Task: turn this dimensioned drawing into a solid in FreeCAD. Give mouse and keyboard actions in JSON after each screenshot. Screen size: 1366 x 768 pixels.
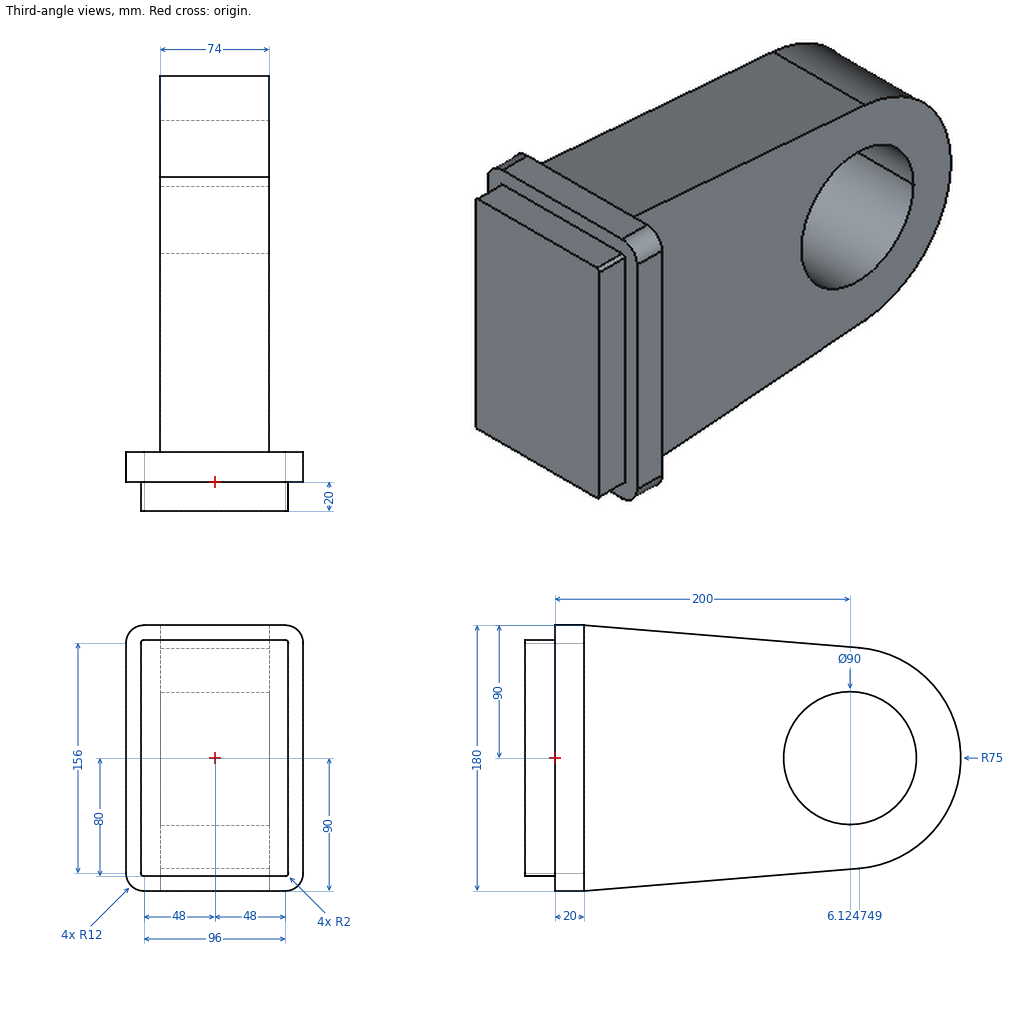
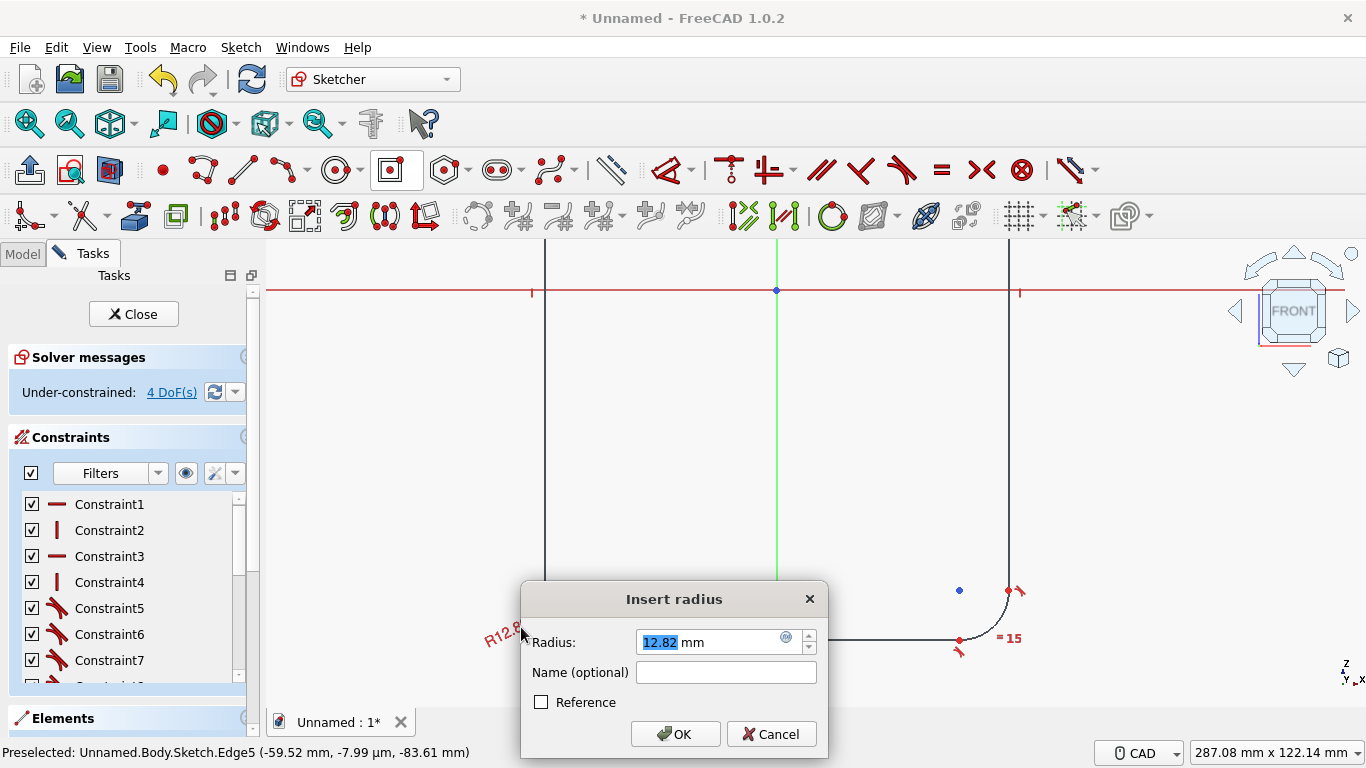
{"action": "type", "text": "12"}
{"action": "key", "text": "Return"}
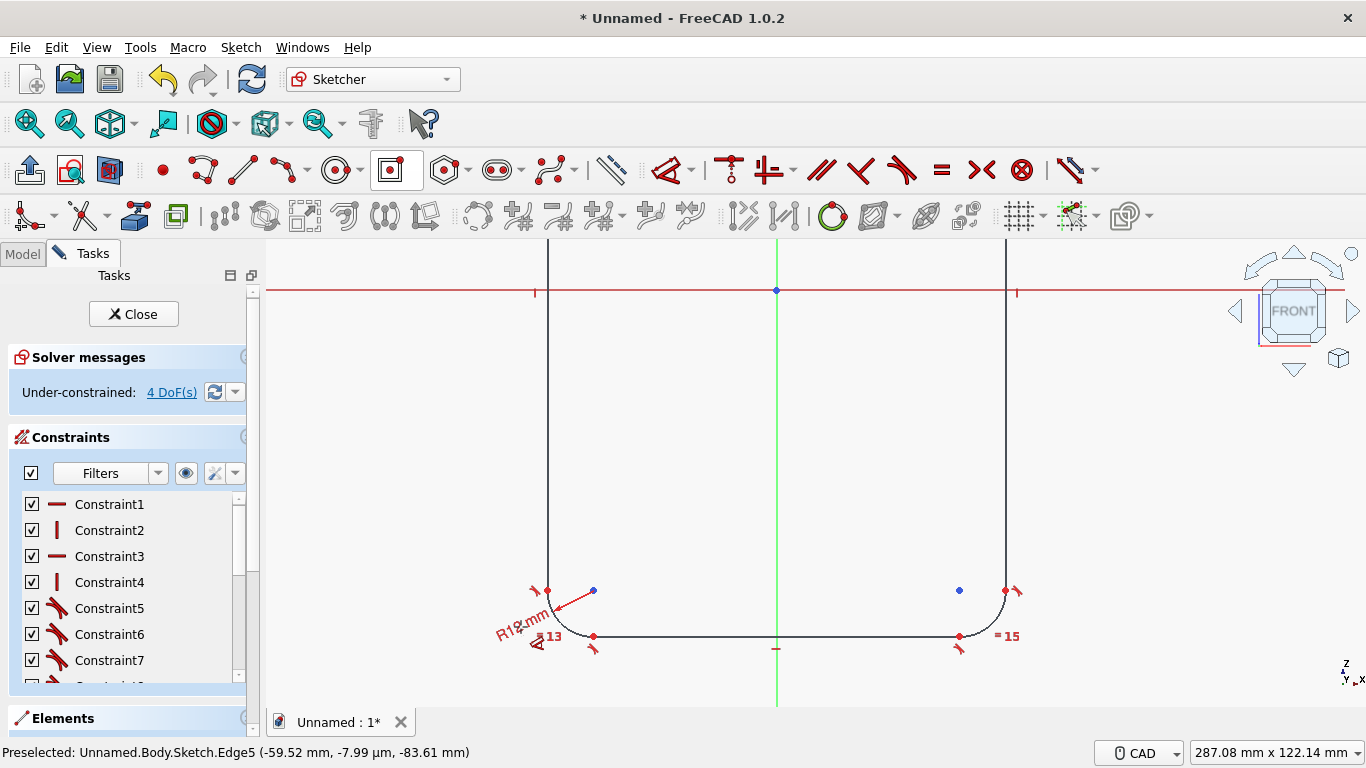
{"action": "left_click", "coordinate": [850, 637]}
{"action": "left_click", "coordinate": [692, 671]}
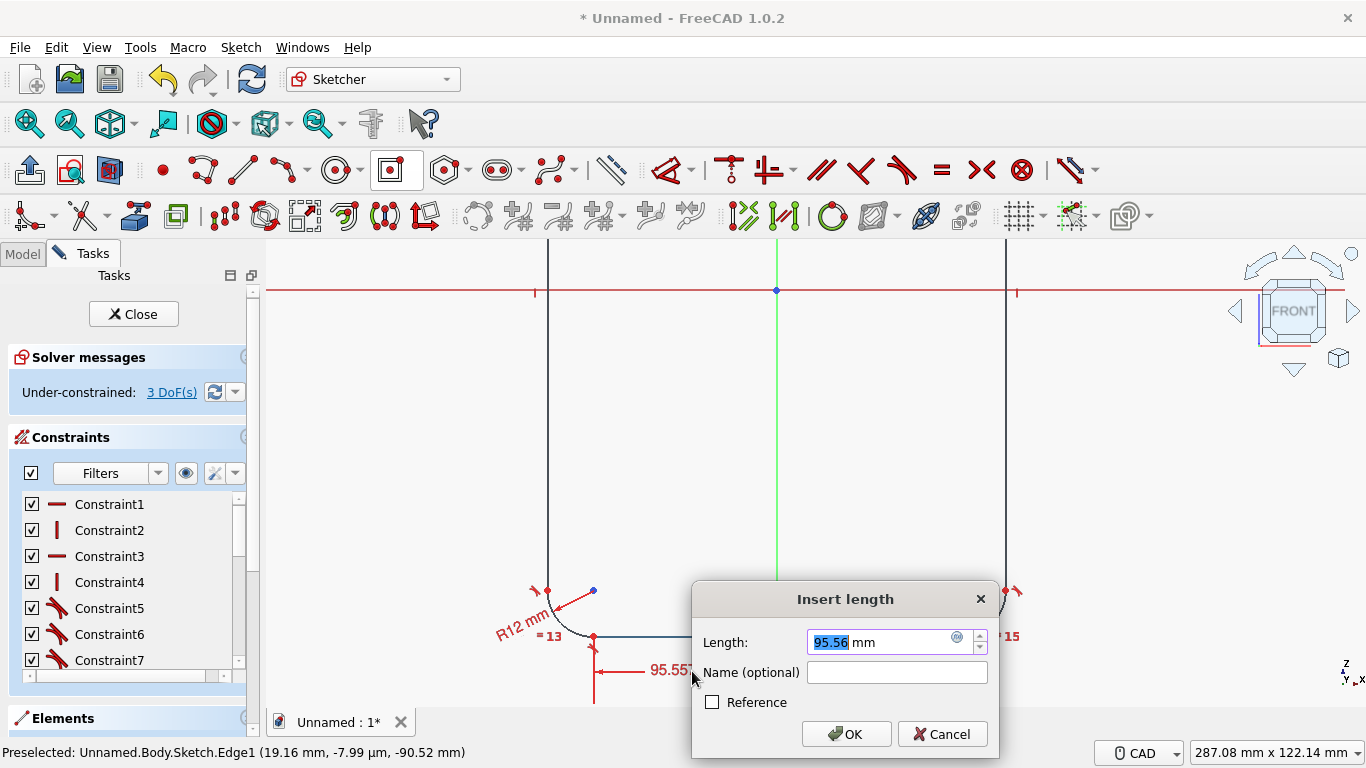
{"action": "type", "text": "96"}
{"action": "key", "text": "Return"}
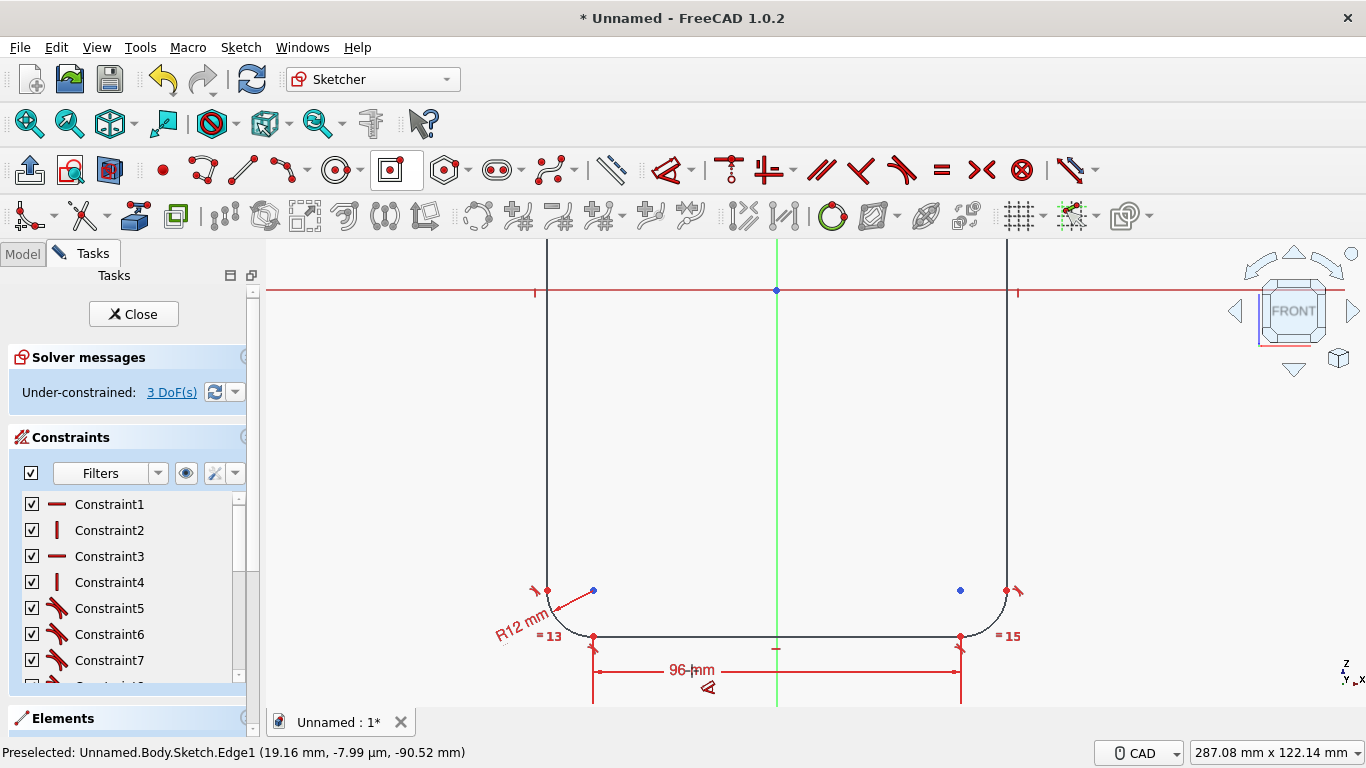
{"action": "left_click", "coordinate": [547, 412]}
{"action": "left_click", "coordinate": [513, 429]}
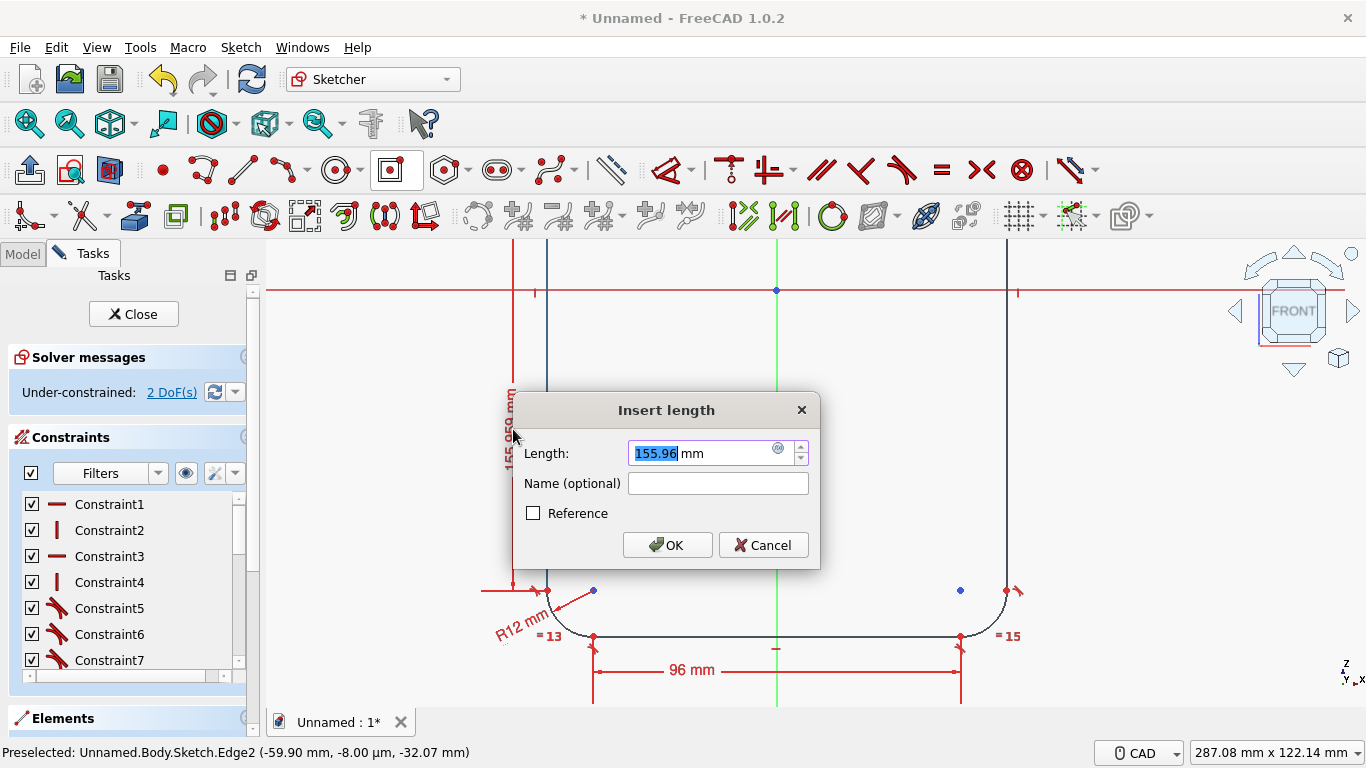
{"action": "type", "text": "156"}
{"action": "key", "text": "Return"}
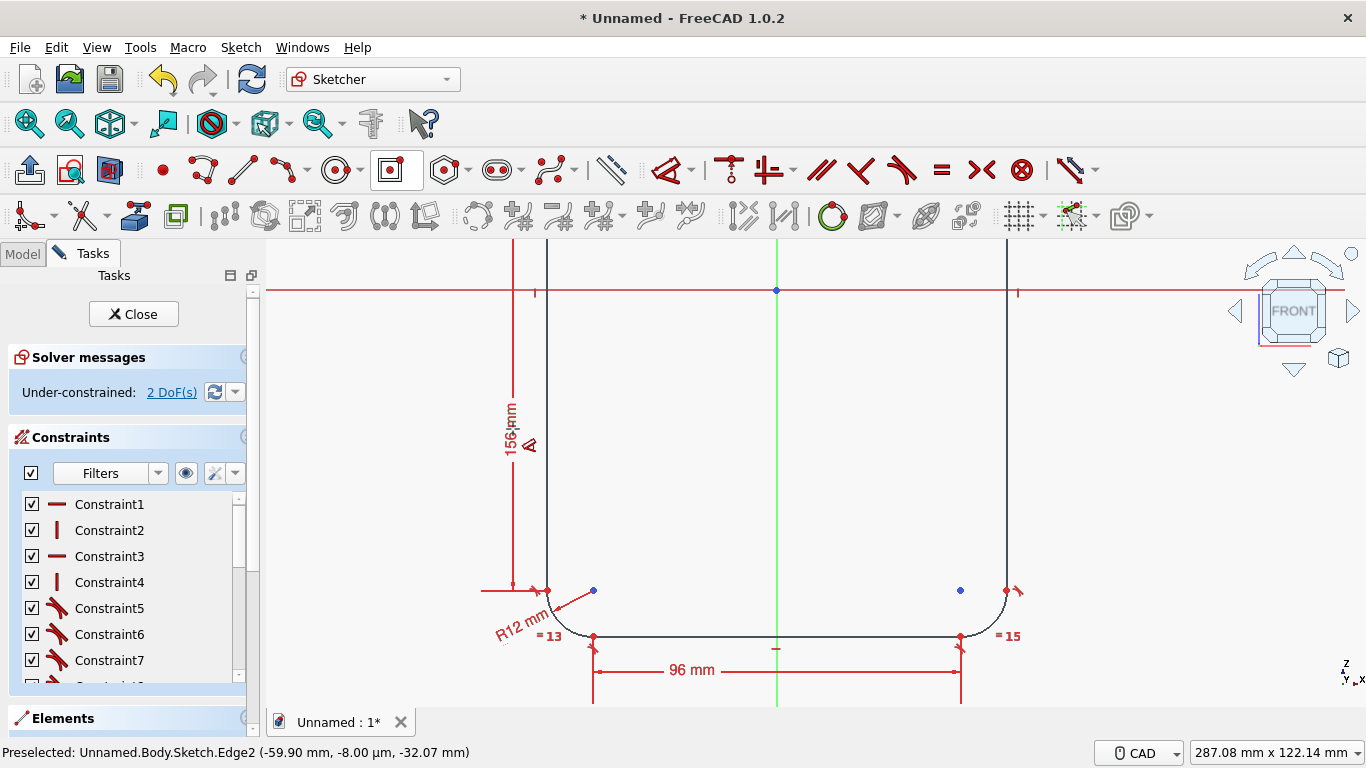
{"action": "left_click", "coordinate": [961, 637]}
{"action": "left_click", "coordinate": [869, 671]}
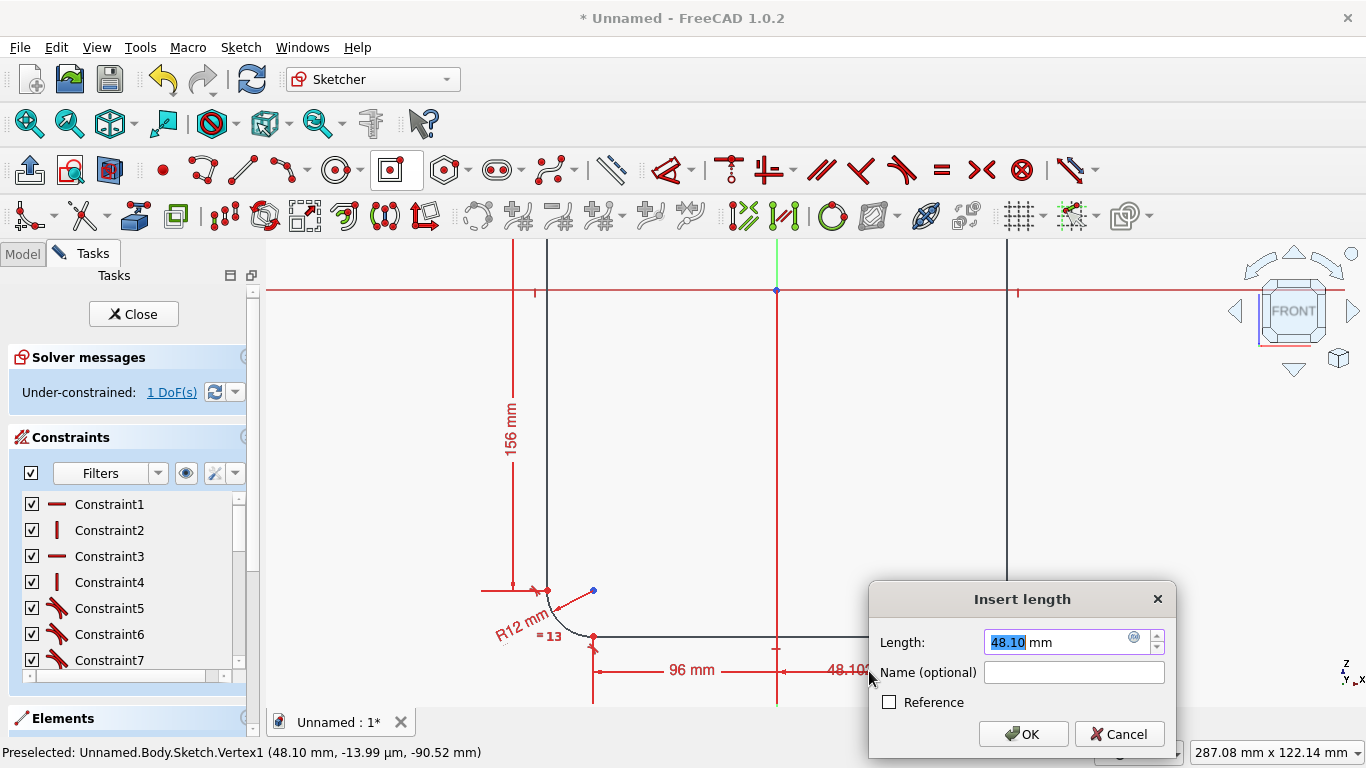
{"action": "type", "text": "48"}
{"action": "key", "text": "Return"}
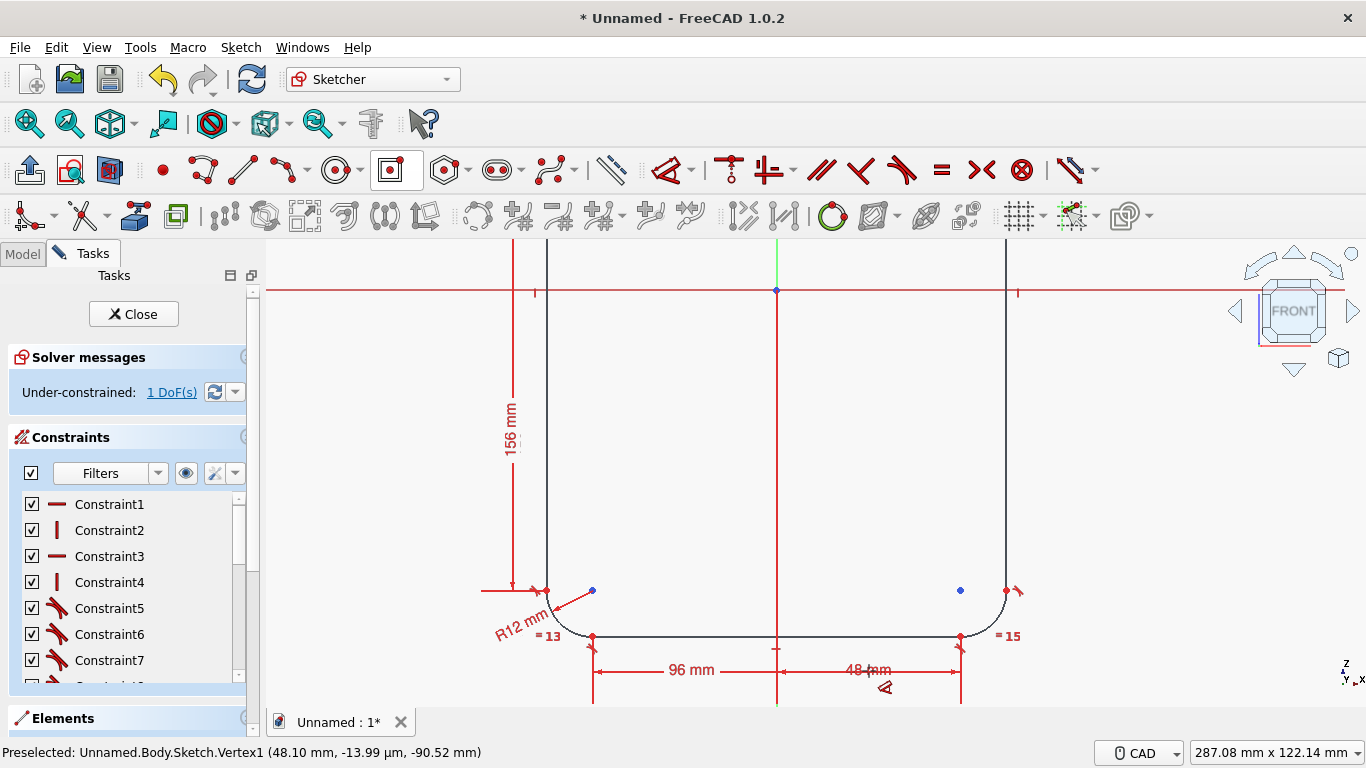
{"action": "left_click", "coordinate": [961, 637]}
{"action": "left_click", "coordinate": [743, 464]}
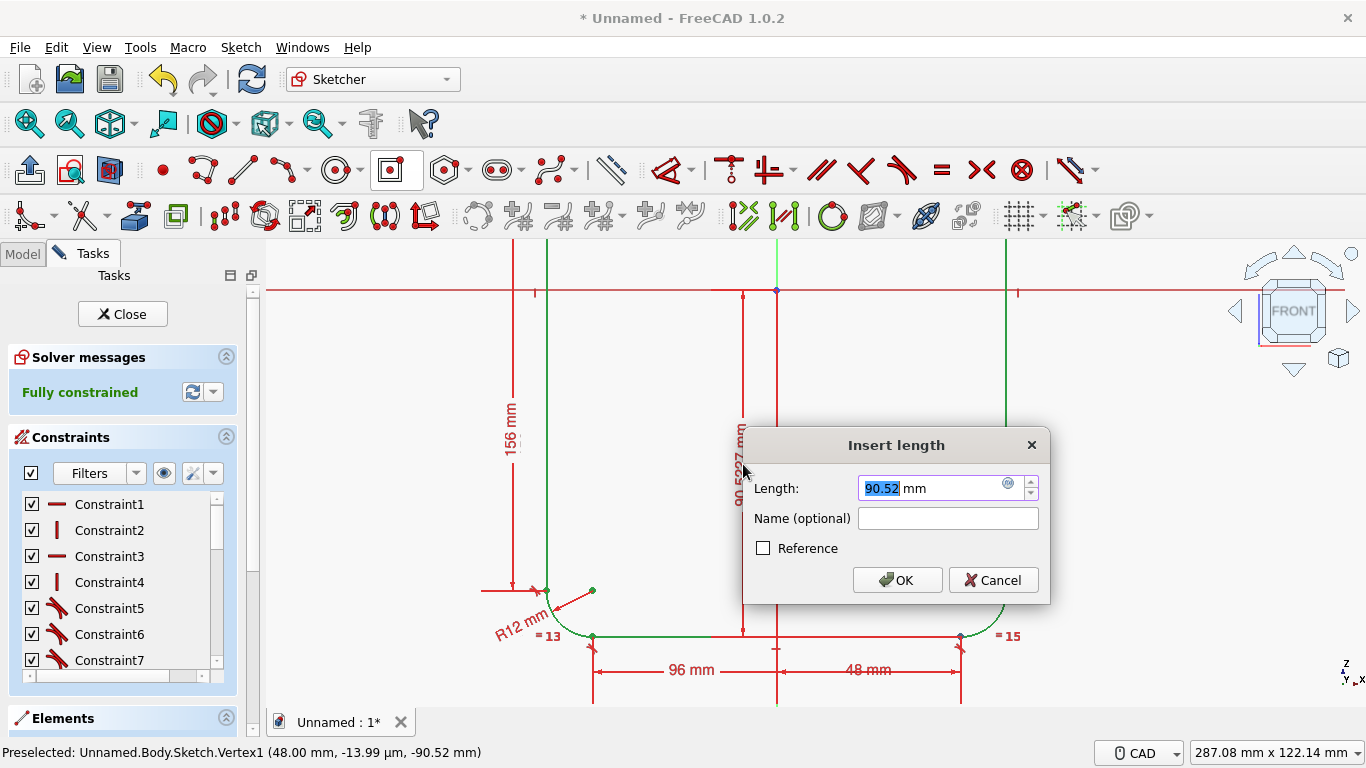
{"action": "type", "text": "90"}
{"action": "key", "text": "Return"}
{"action": "key", "text": "Escape"}